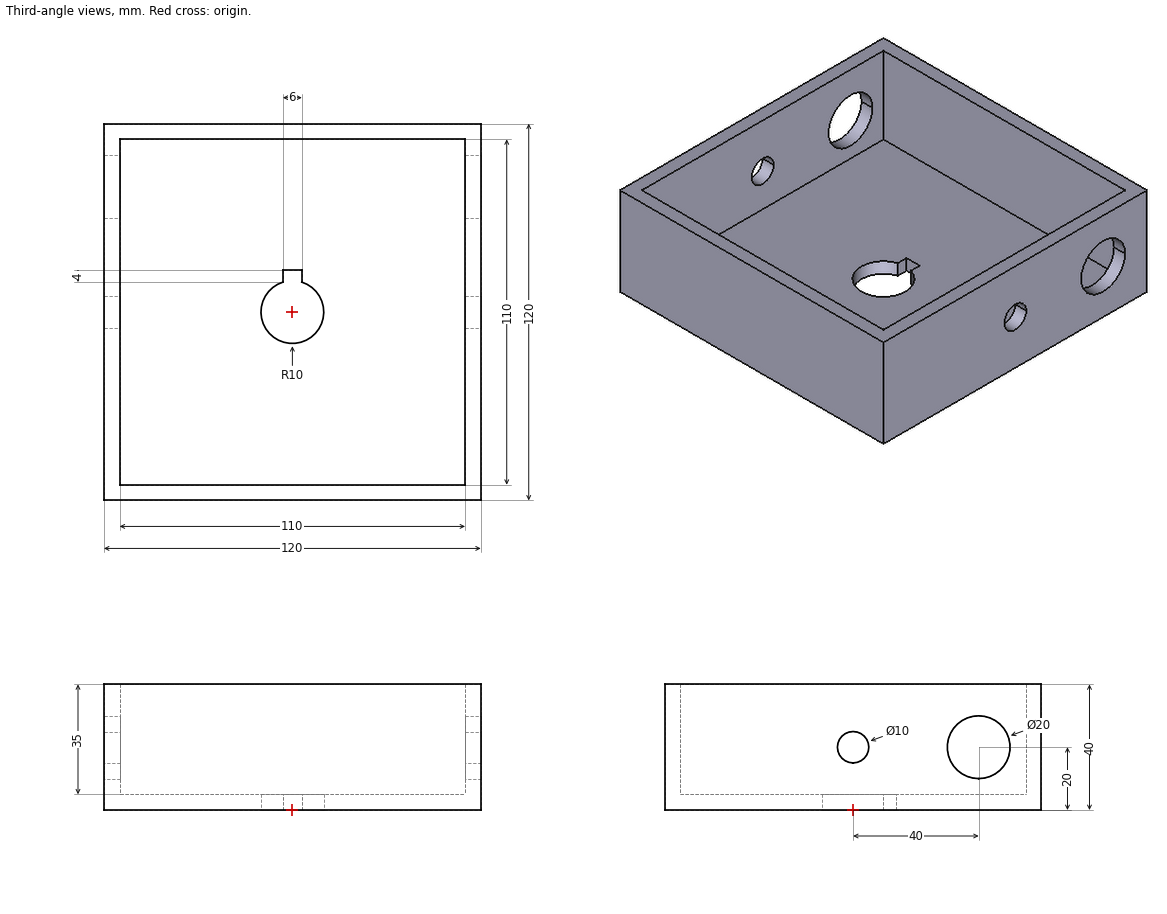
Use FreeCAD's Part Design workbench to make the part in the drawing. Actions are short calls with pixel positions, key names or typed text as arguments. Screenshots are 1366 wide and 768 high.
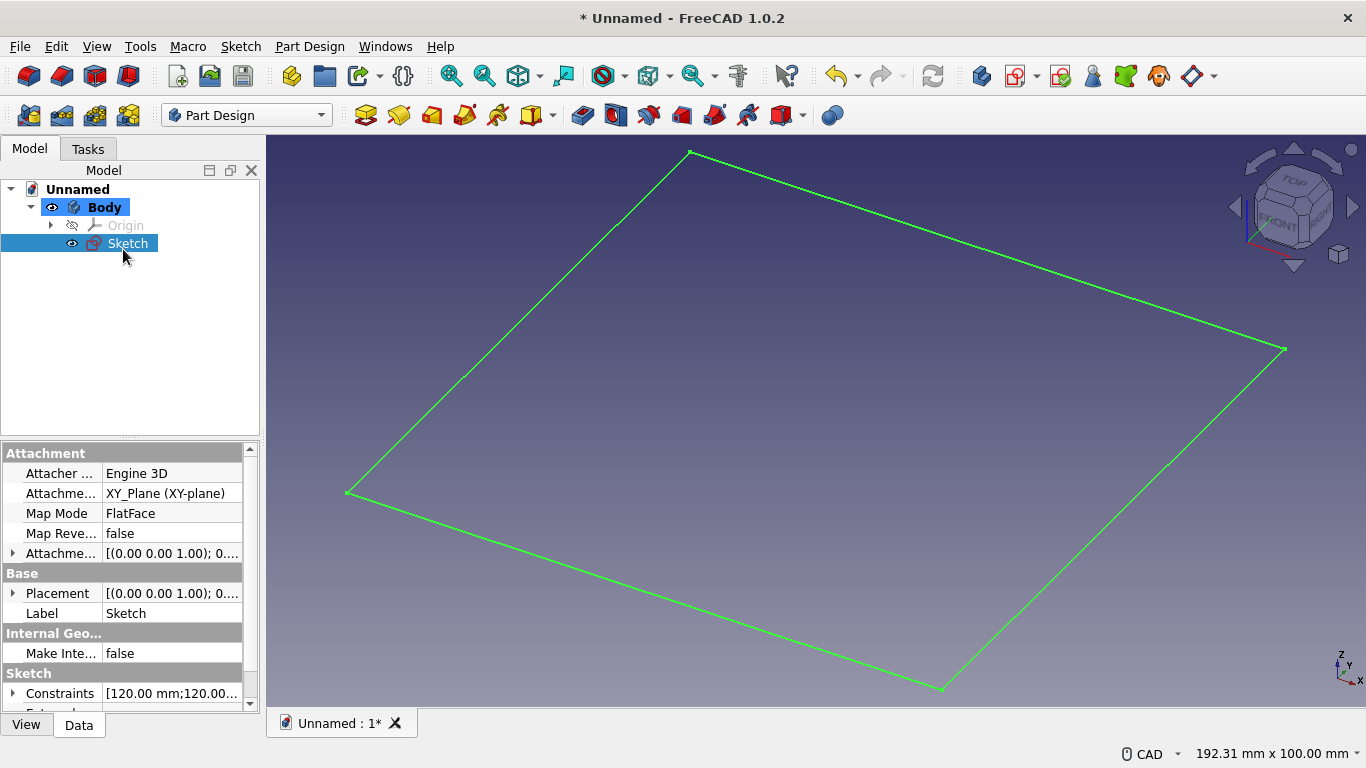
click(366, 116)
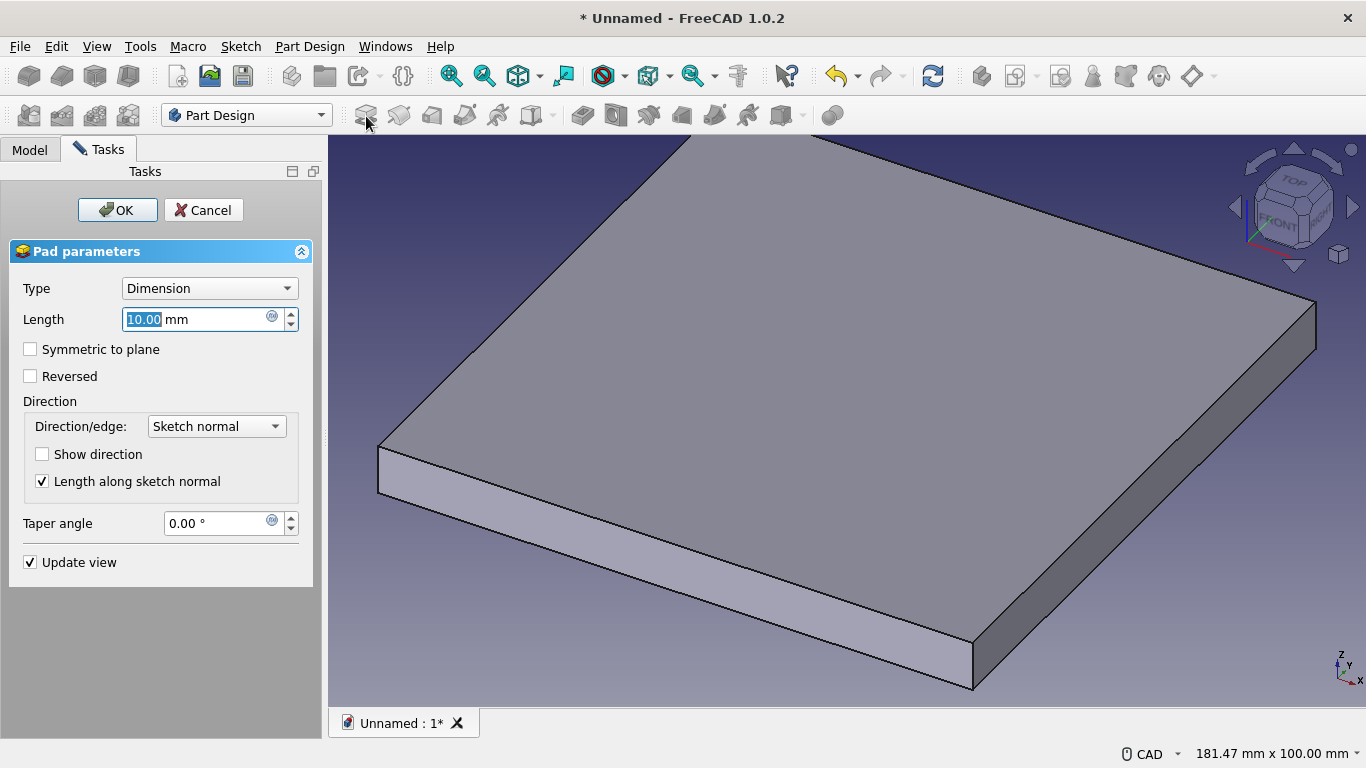
text(40)
key(Tab)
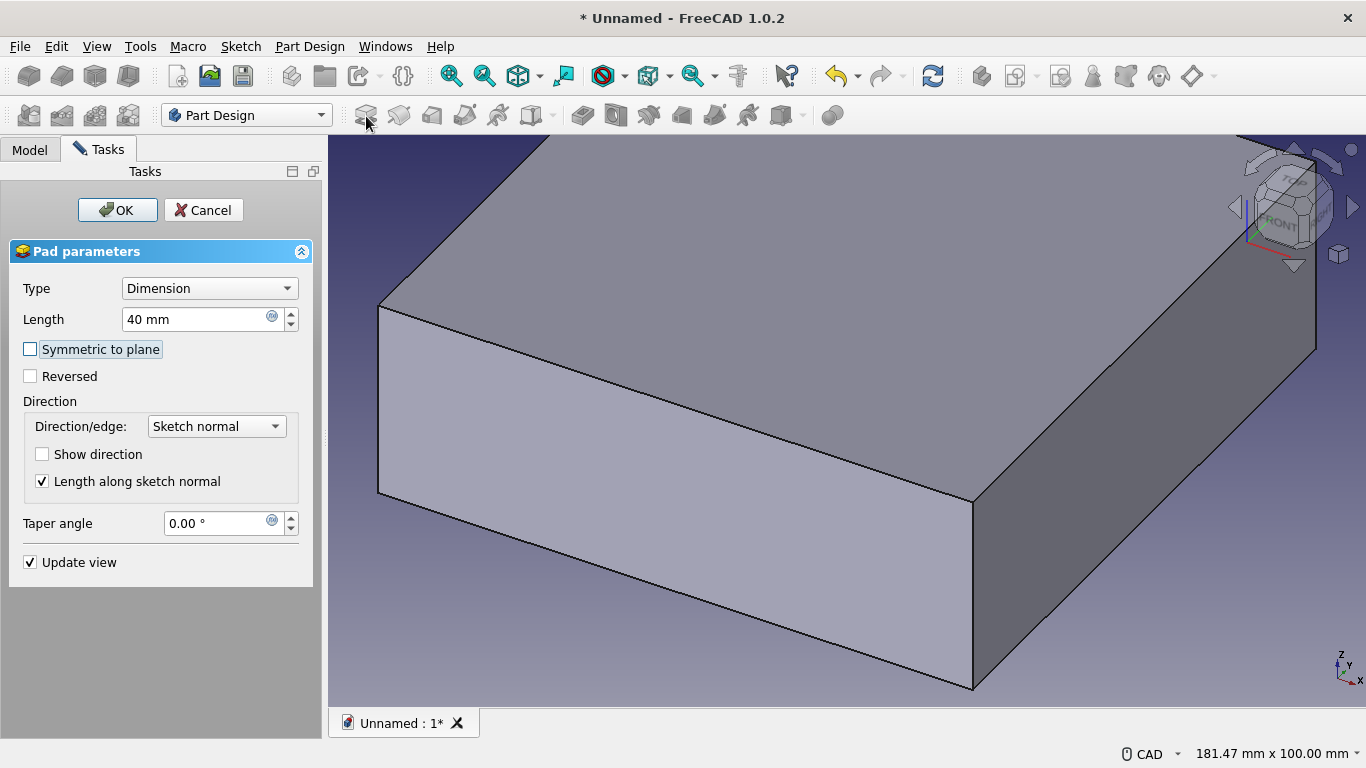
click(118, 210)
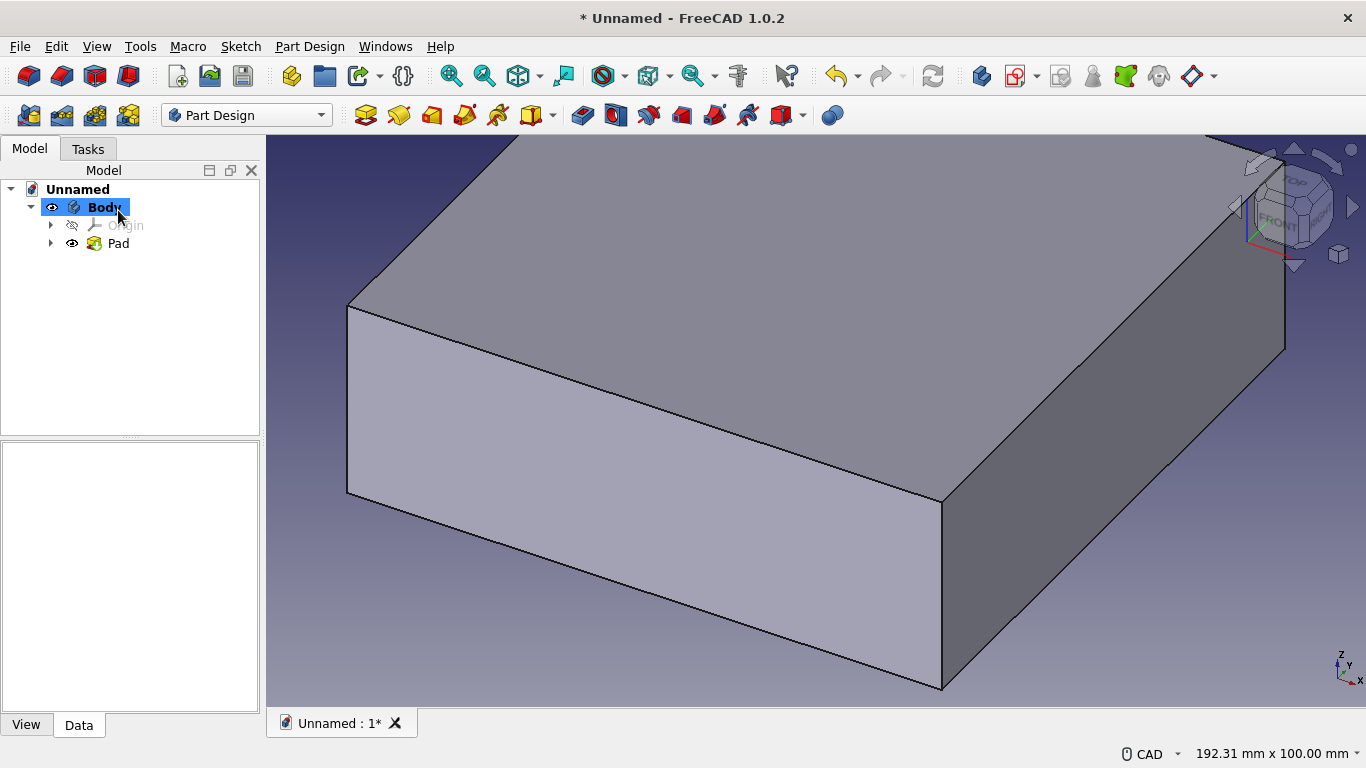
key(v)
key(f)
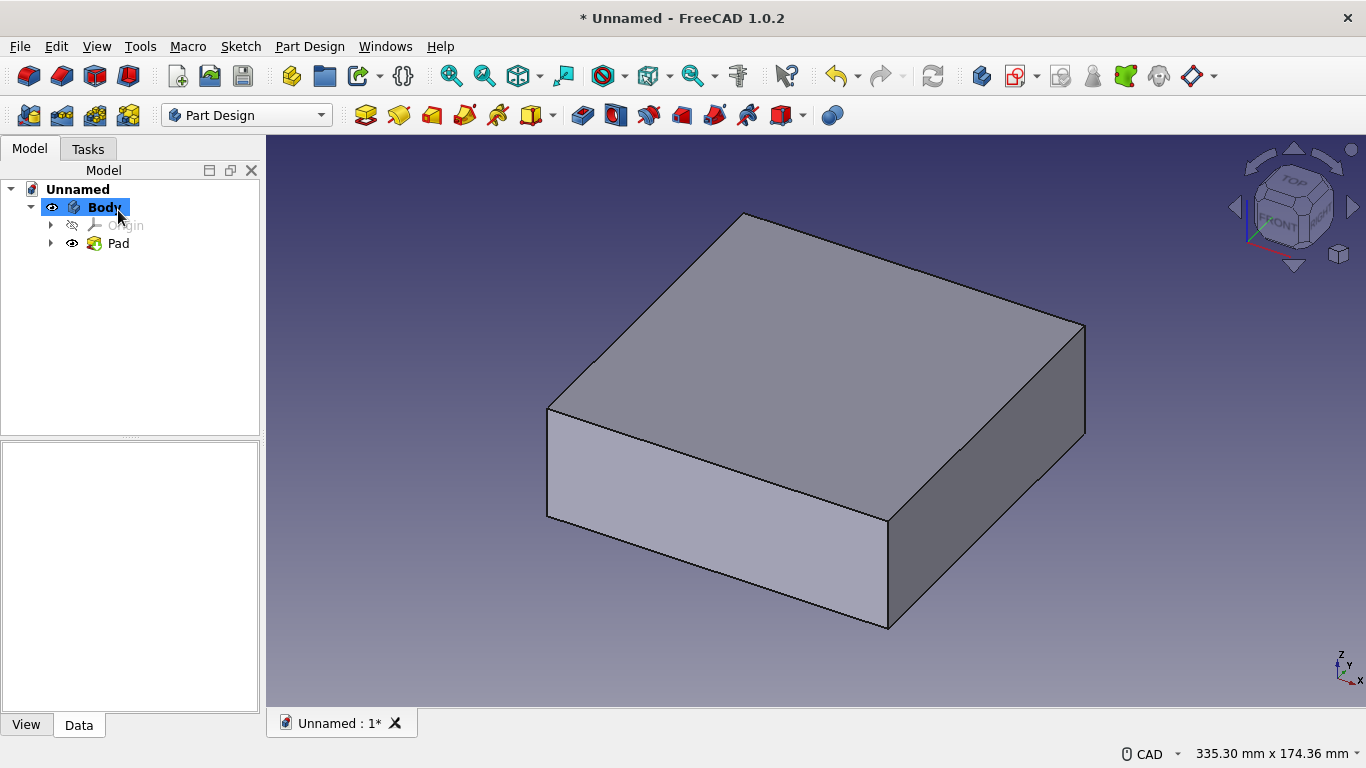
click(1043, 421)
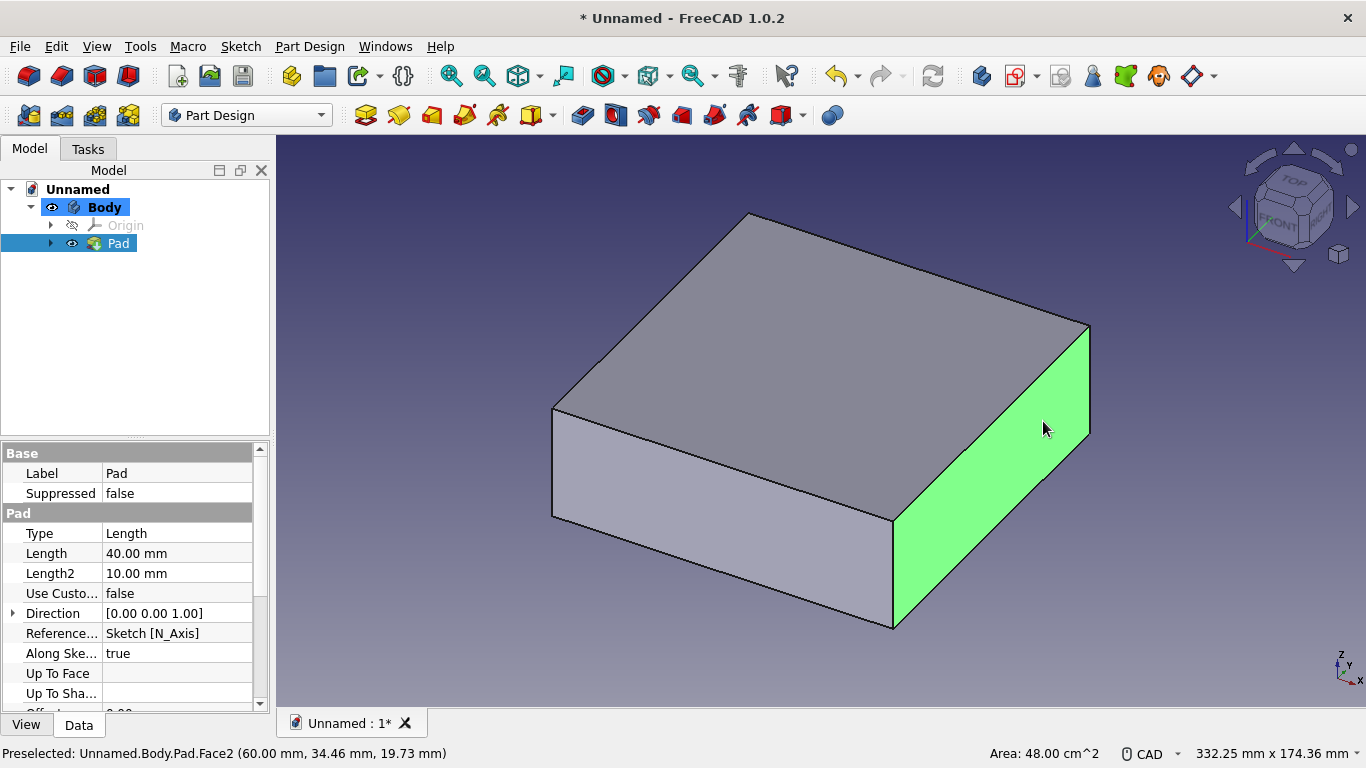
click(1014, 76)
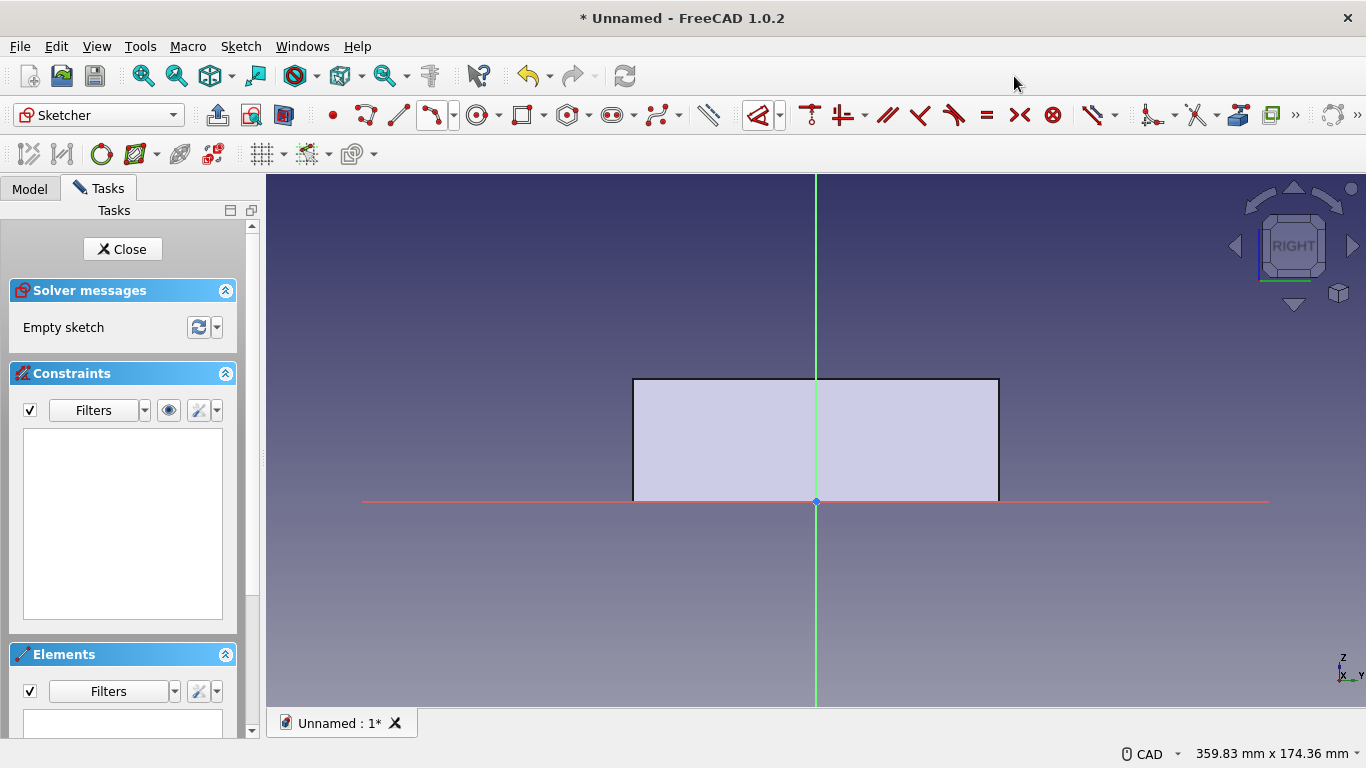
scroll(930, 461, up, 7)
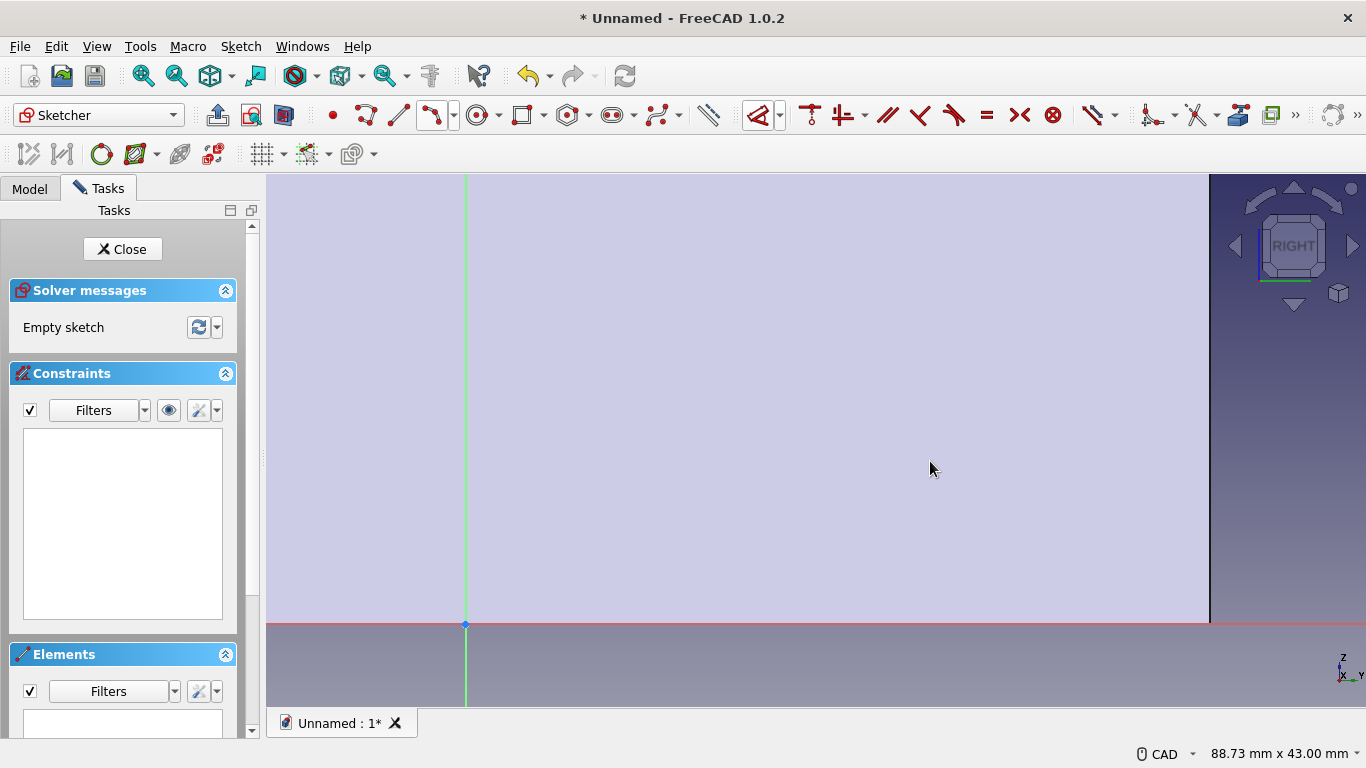
key(g)
key(c)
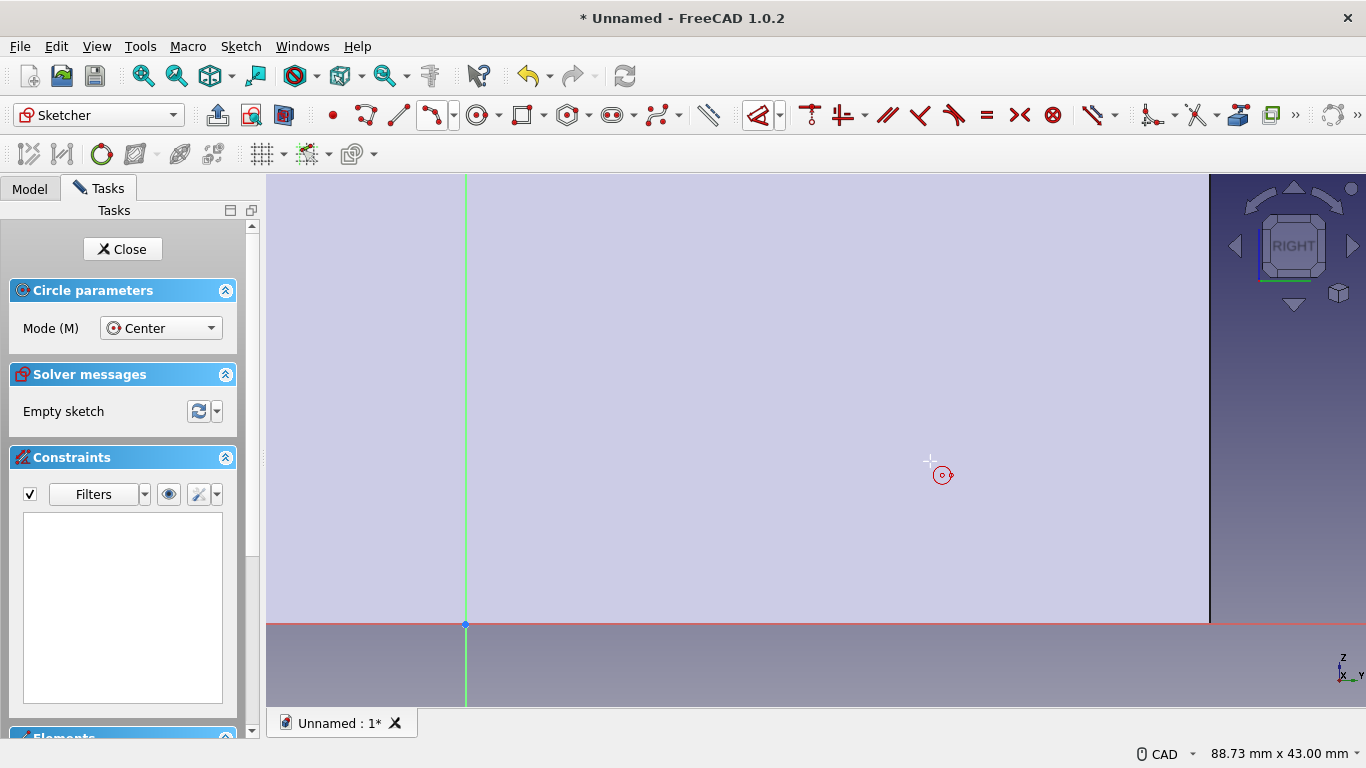
click(962, 376)
move(1049, 289)